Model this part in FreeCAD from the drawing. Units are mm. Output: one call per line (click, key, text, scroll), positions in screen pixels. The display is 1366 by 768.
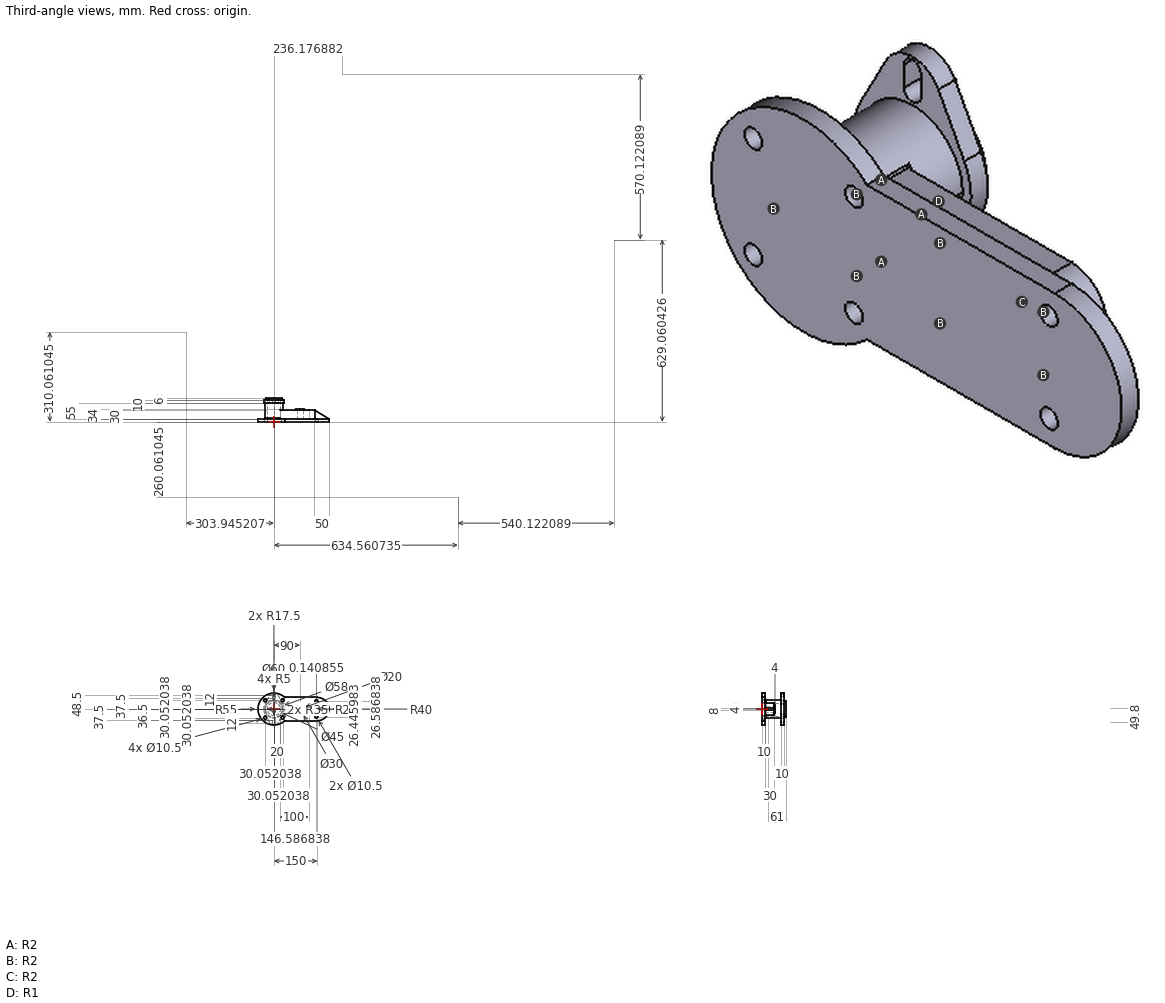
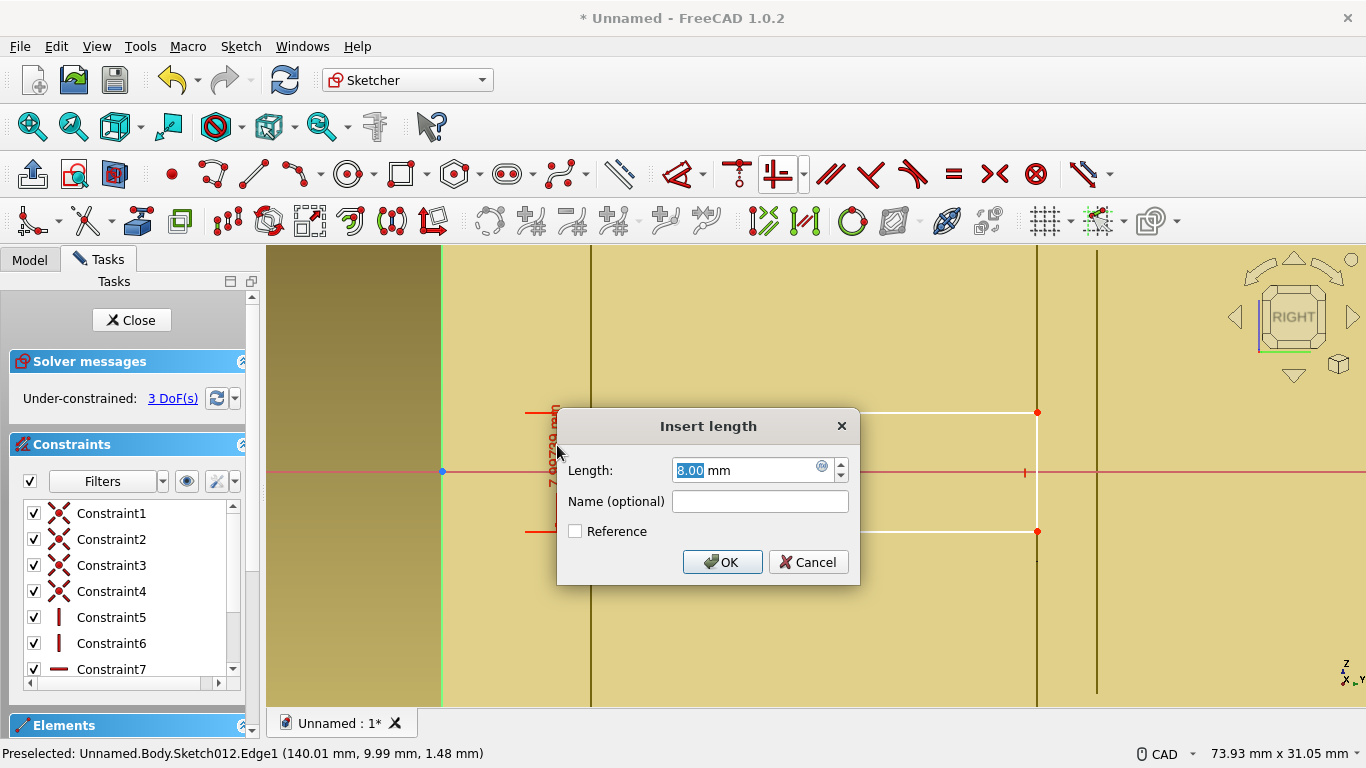
text(8)
key(Return)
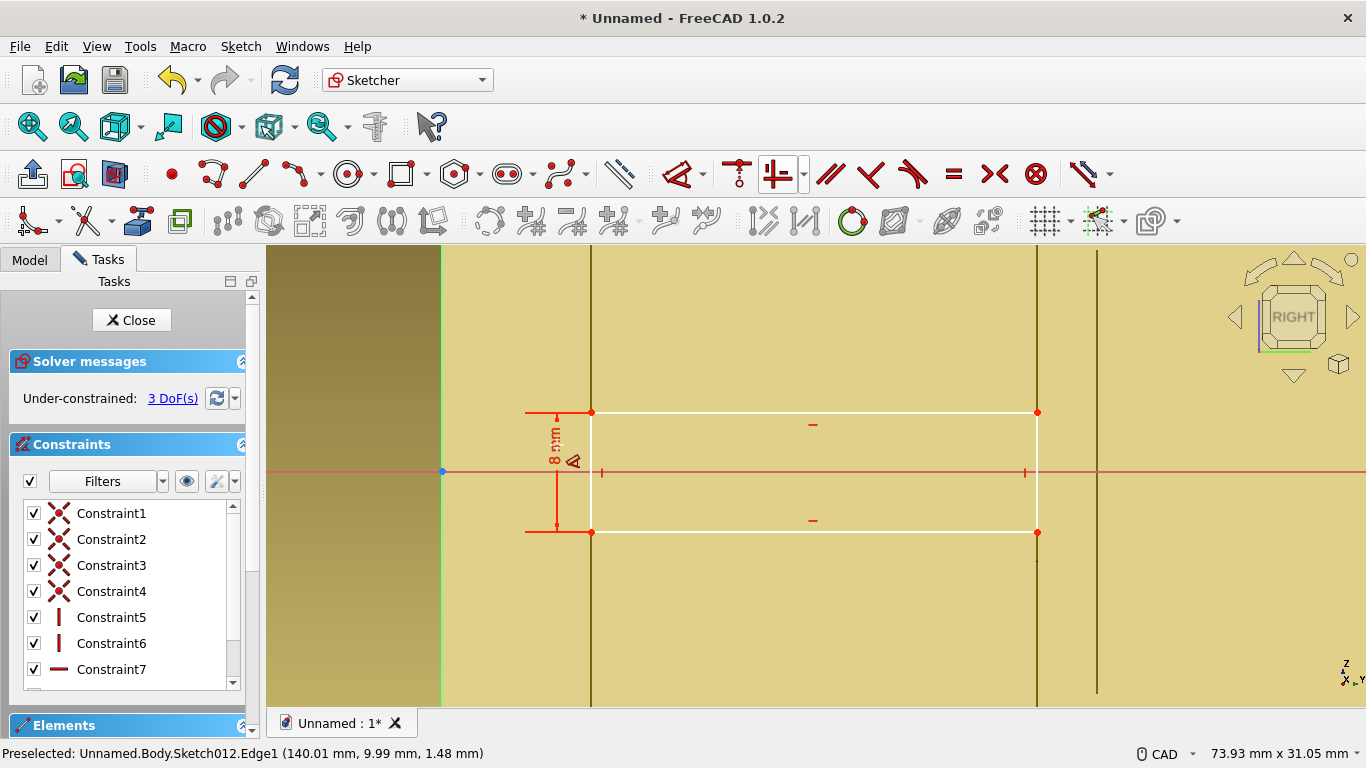
click(725, 532)
click(814, 566)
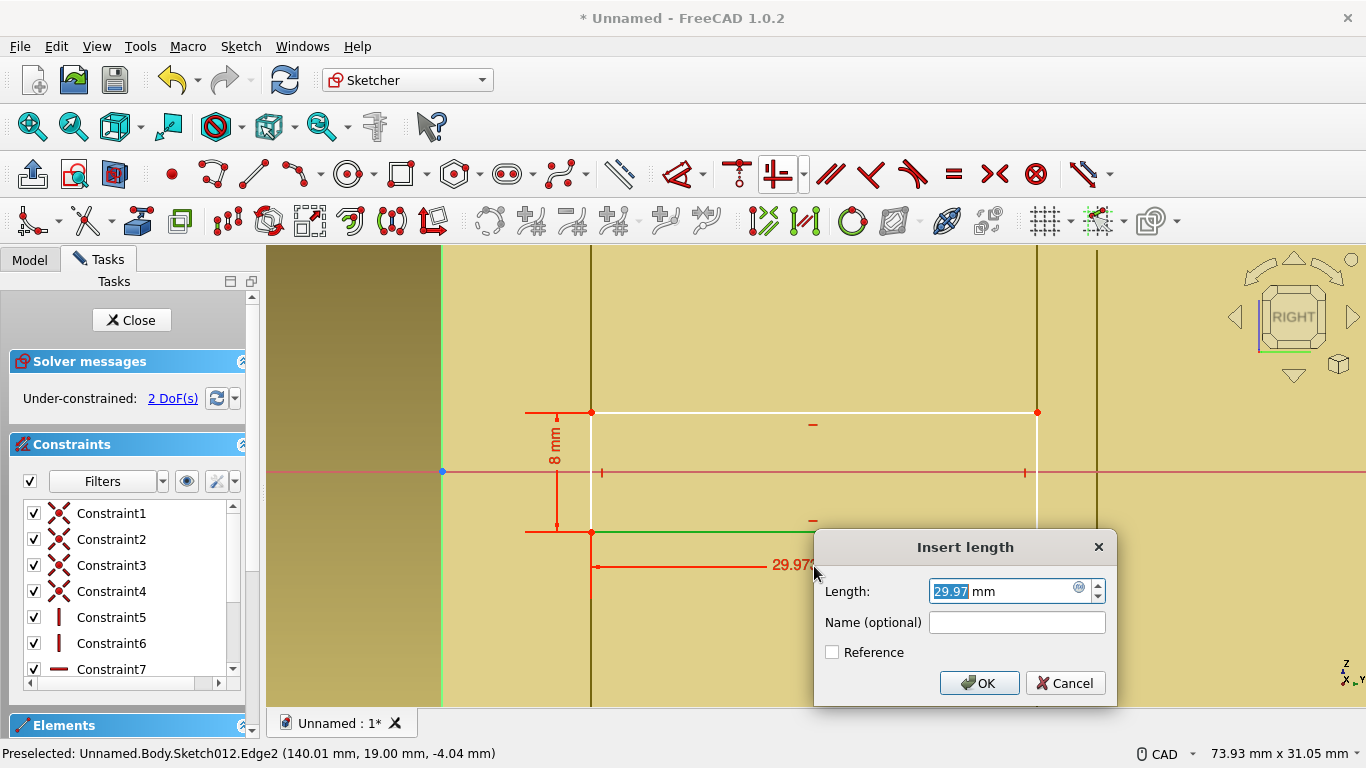
text(30)
key(Return)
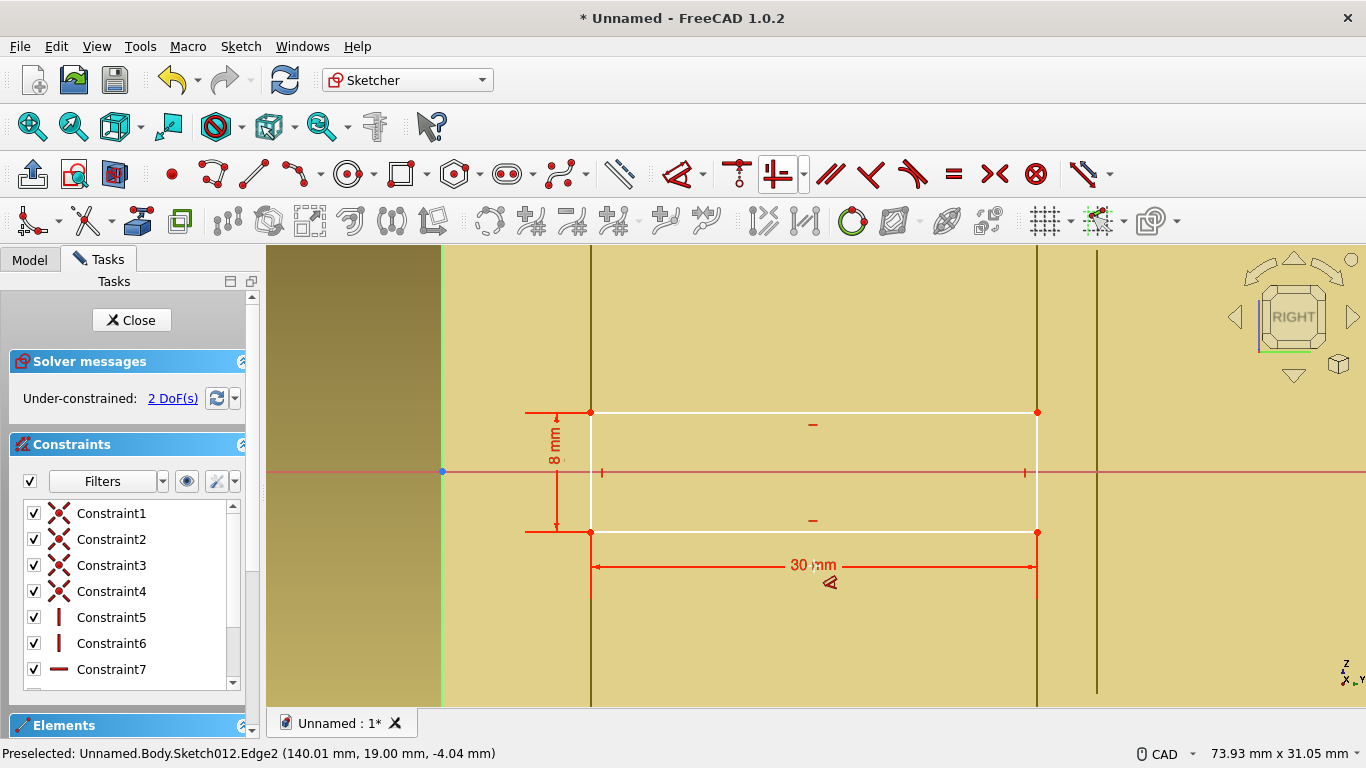
click(591, 413)
click(408, 442)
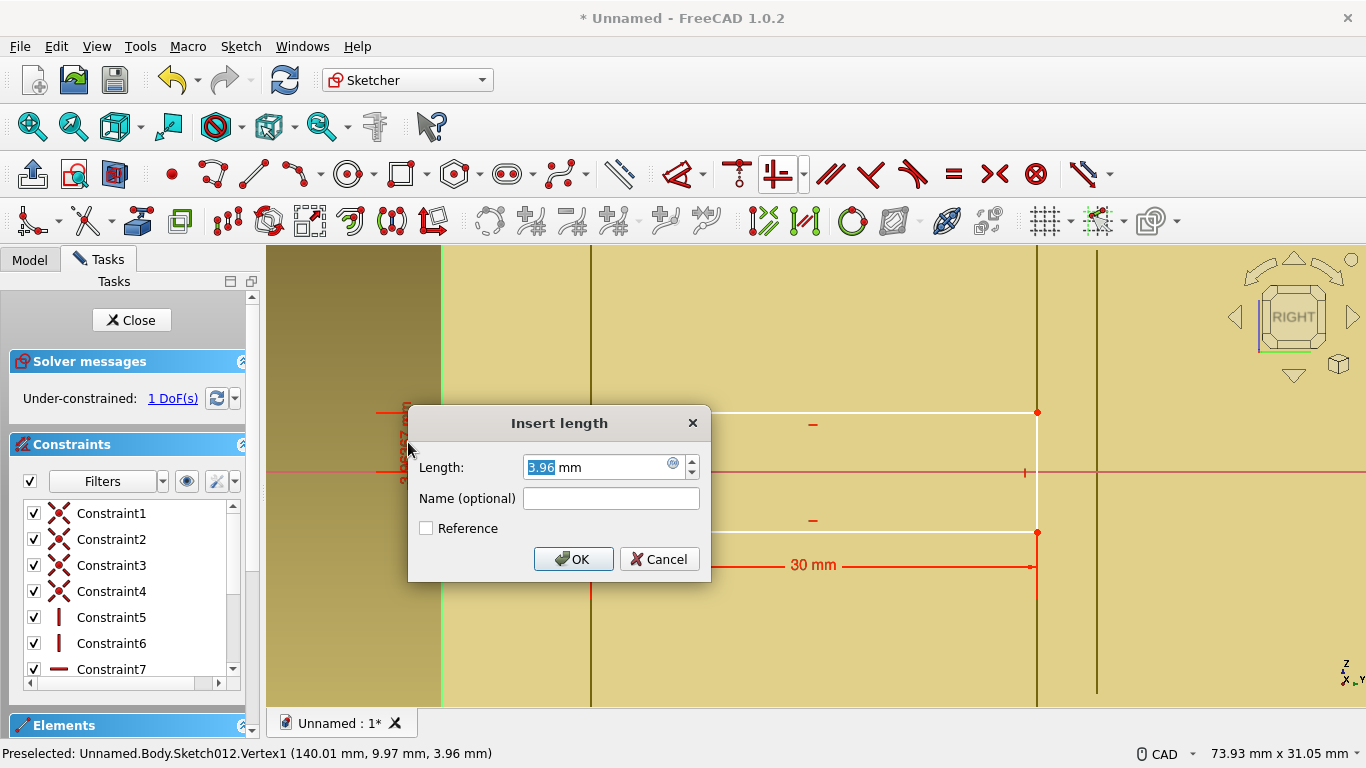
text(4)
key(Return)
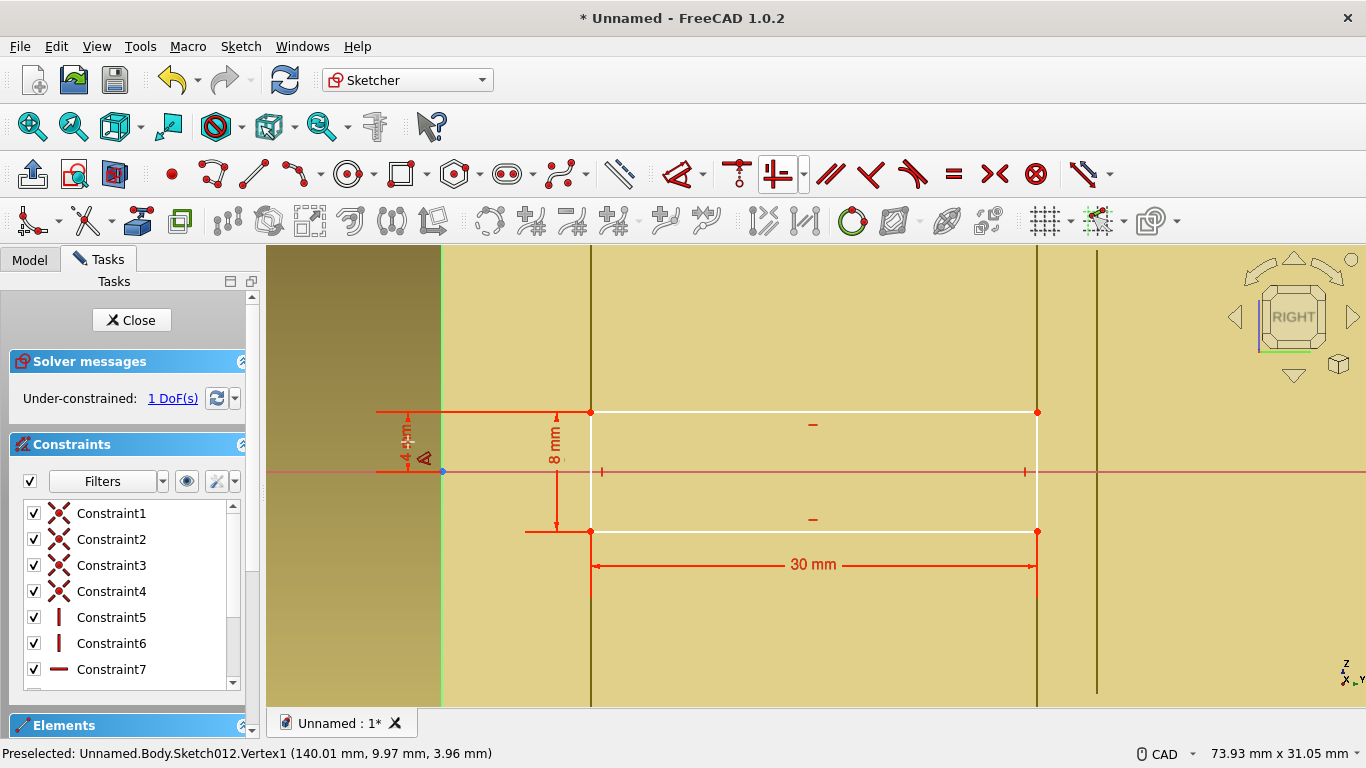
click(591, 412)
click(516, 378)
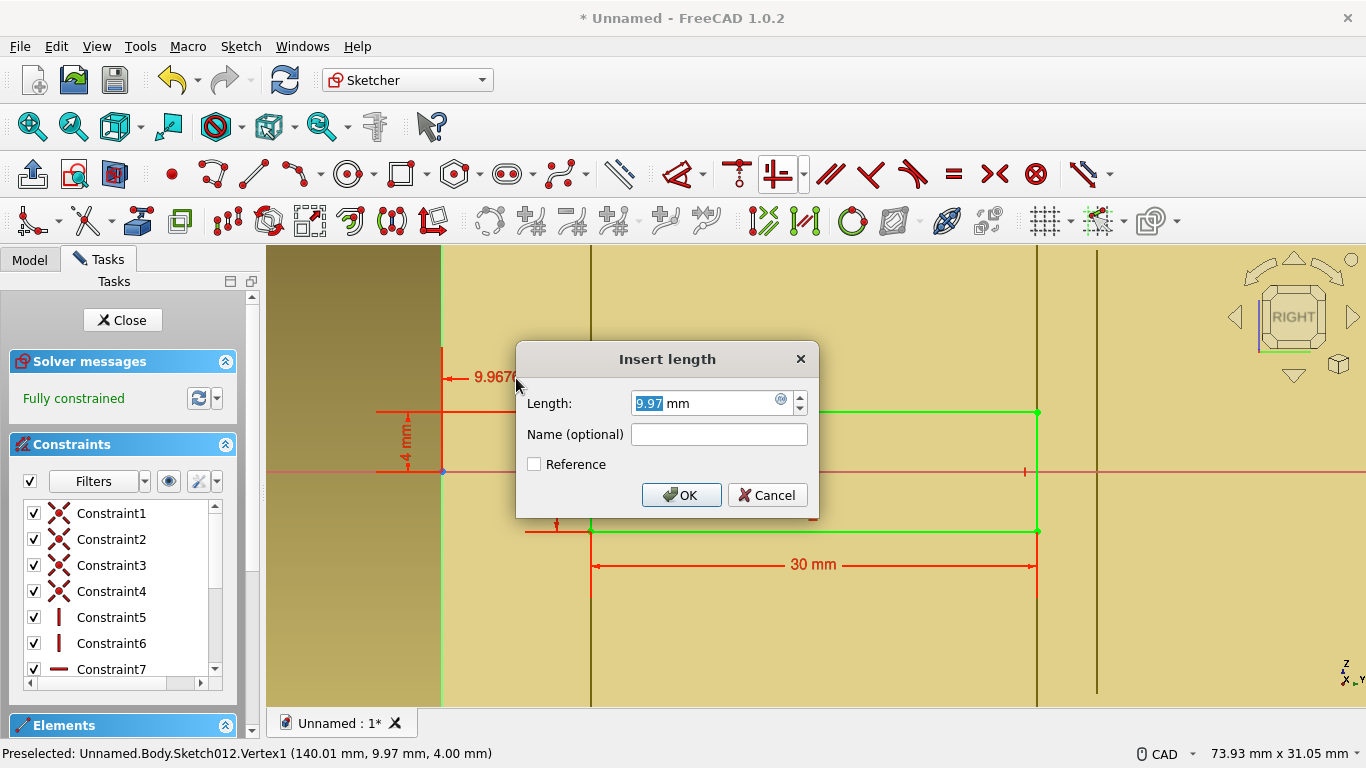
text(10)
key(Return)
key(Escape)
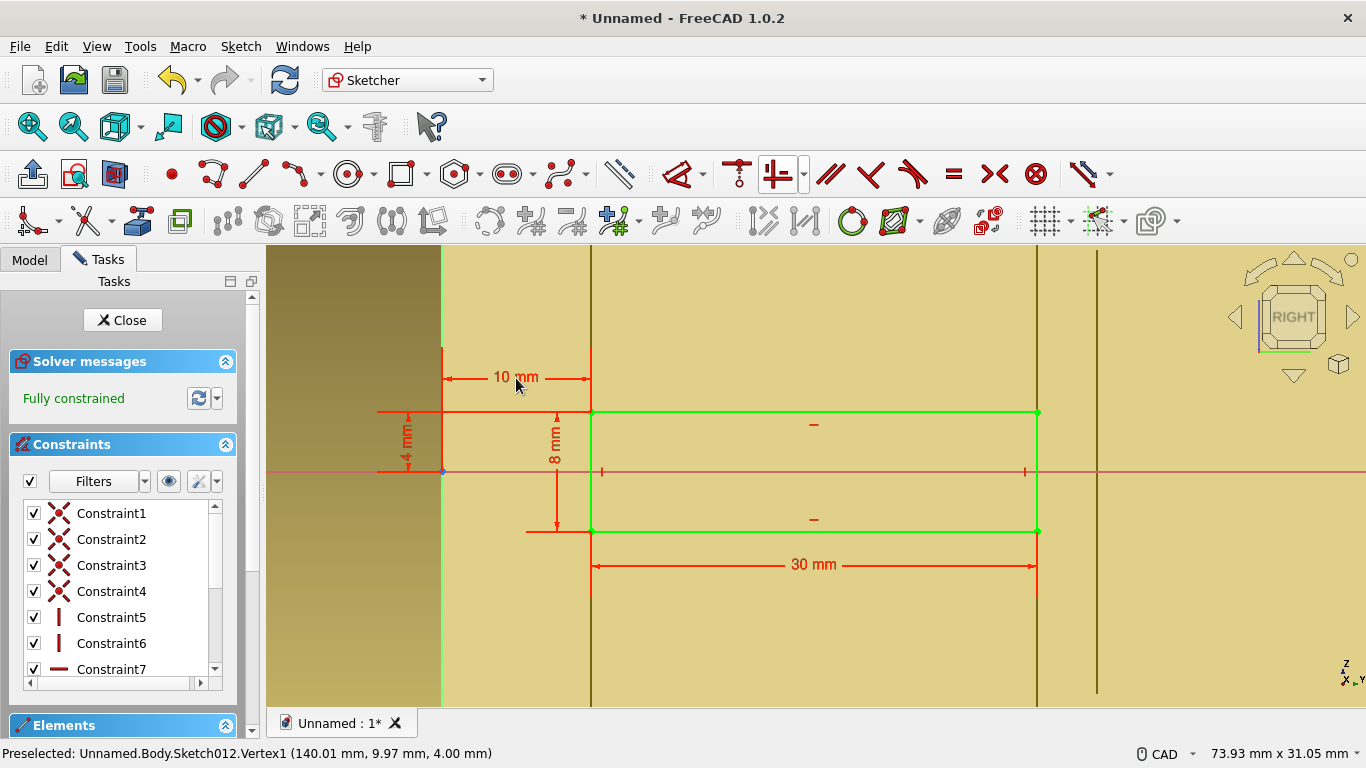
click(123, 320)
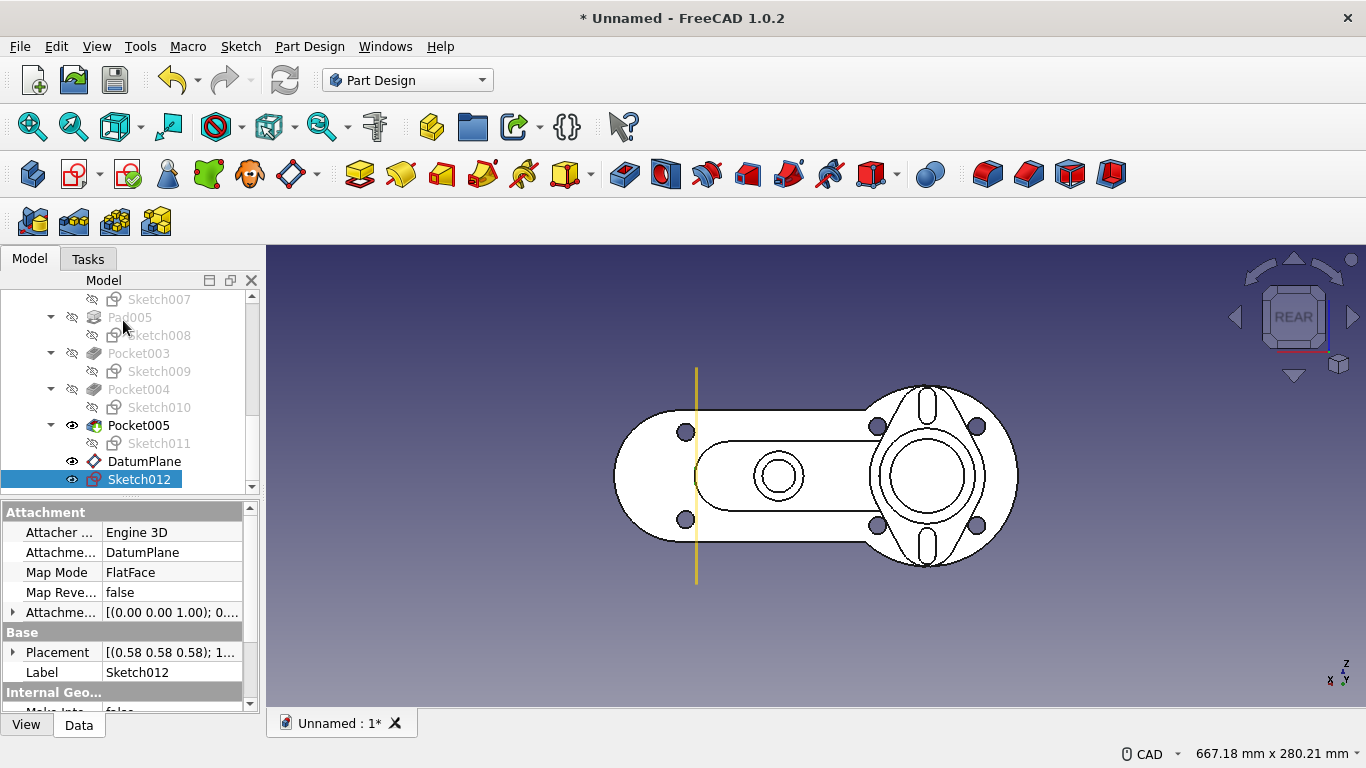
click(360, 174)